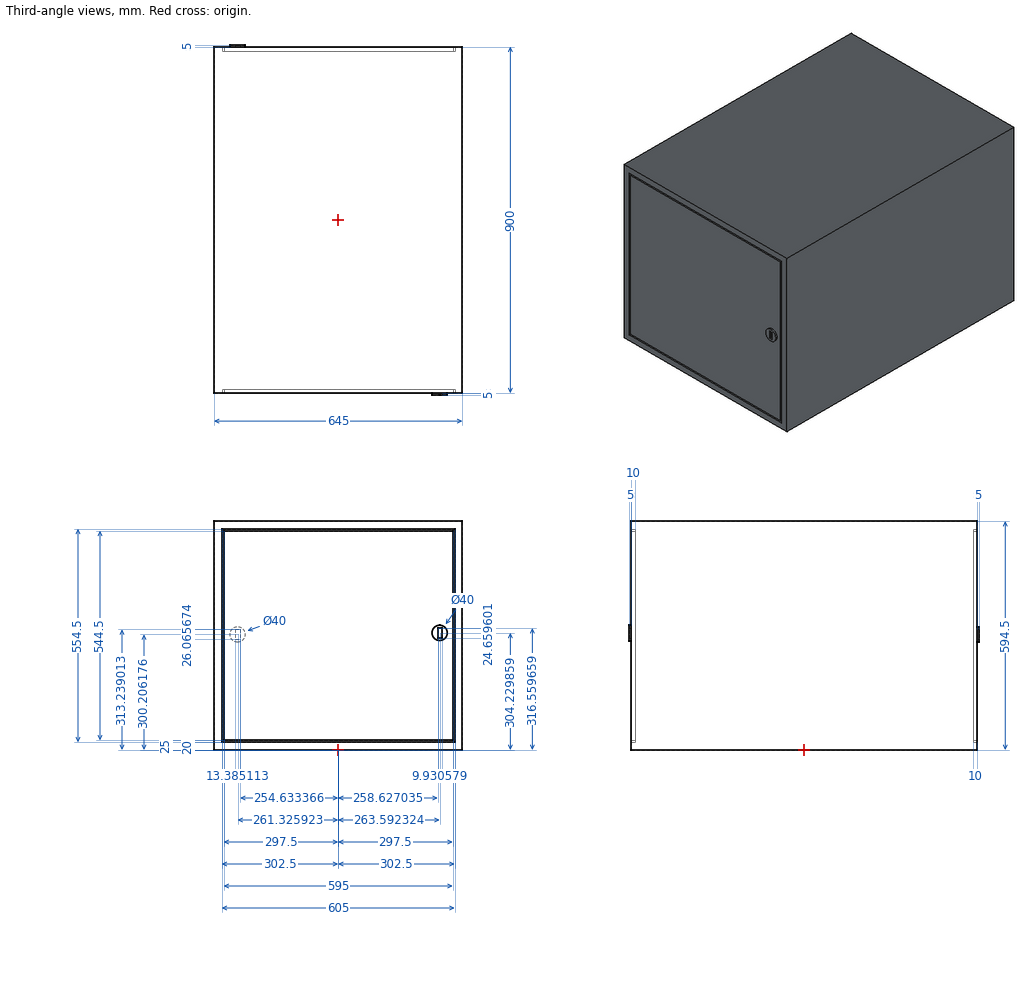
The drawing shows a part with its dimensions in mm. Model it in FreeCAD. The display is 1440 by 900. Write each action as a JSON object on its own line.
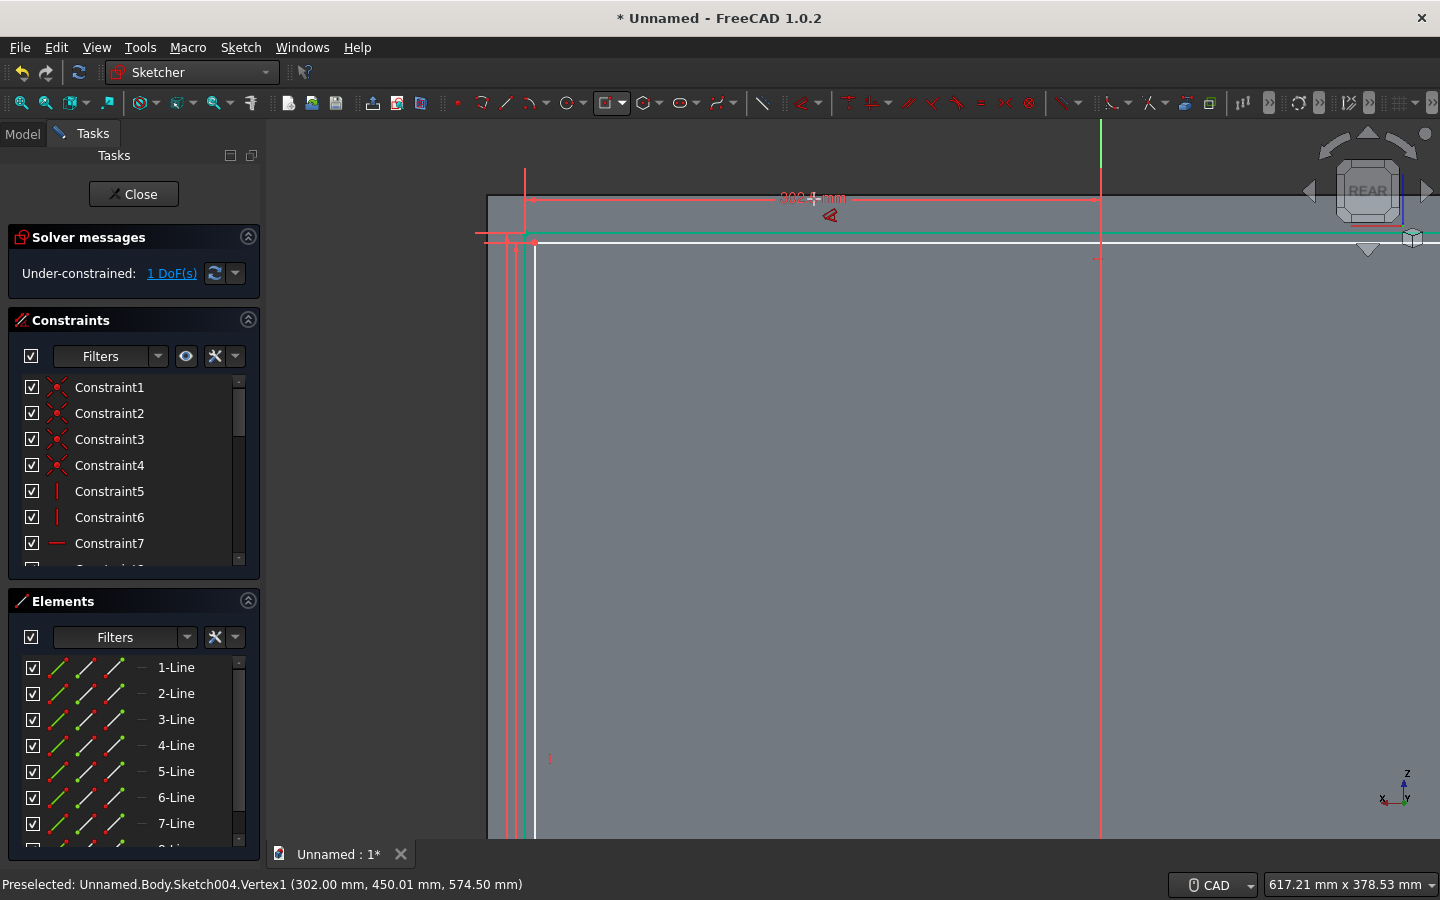
{"action": "left_click", "coordinate": [535, 243]}
{"action": "left_click", "coordinate": [688, 209]}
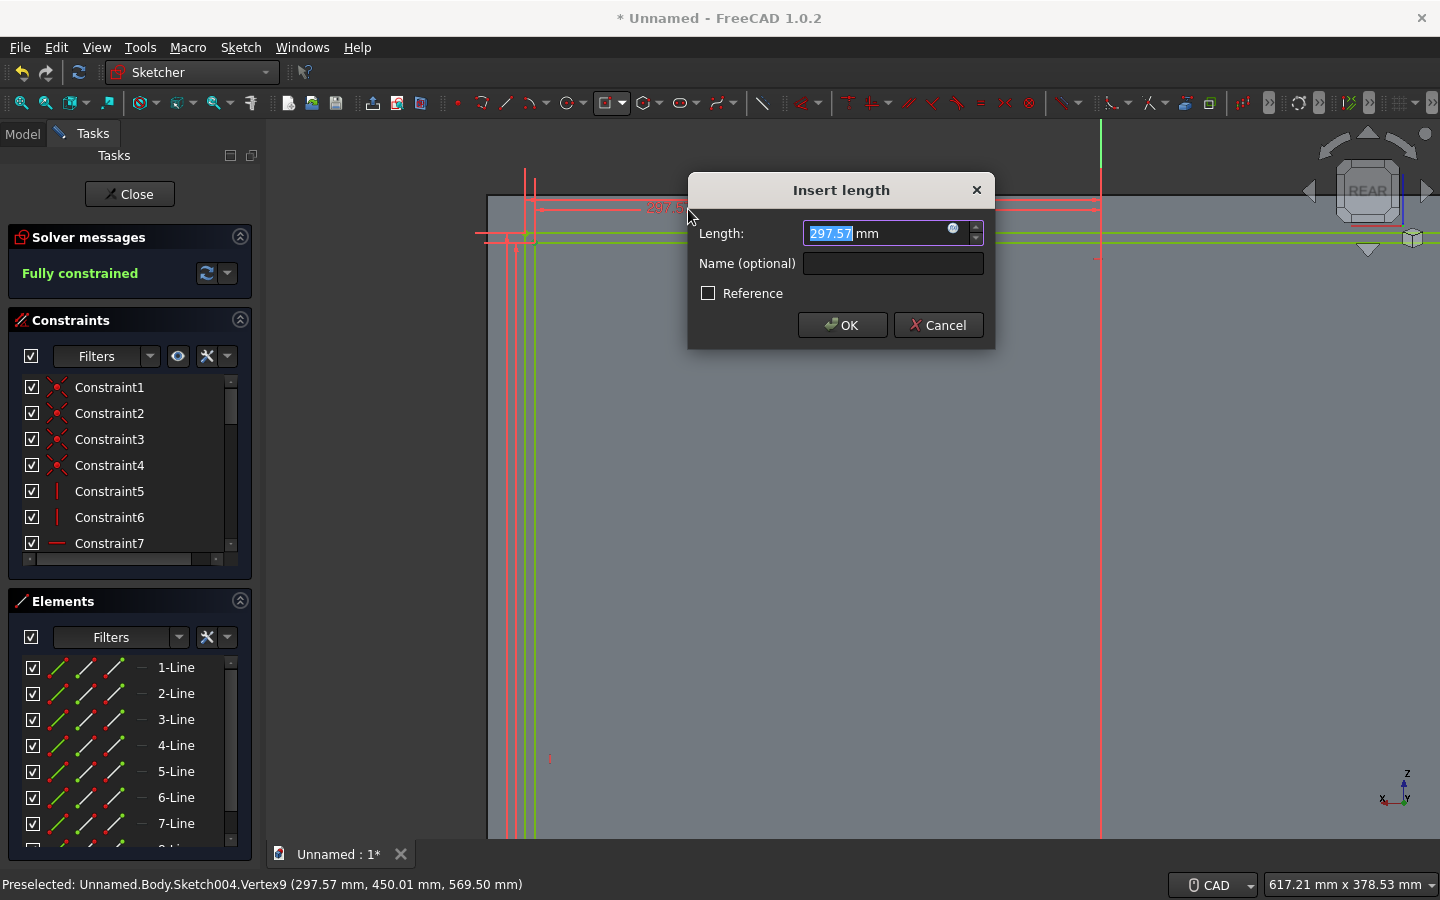
{"action": "type", "text": "297.5"}
{"action": "key", "text": "Return"}
{"action": "key", "text": "Escape"}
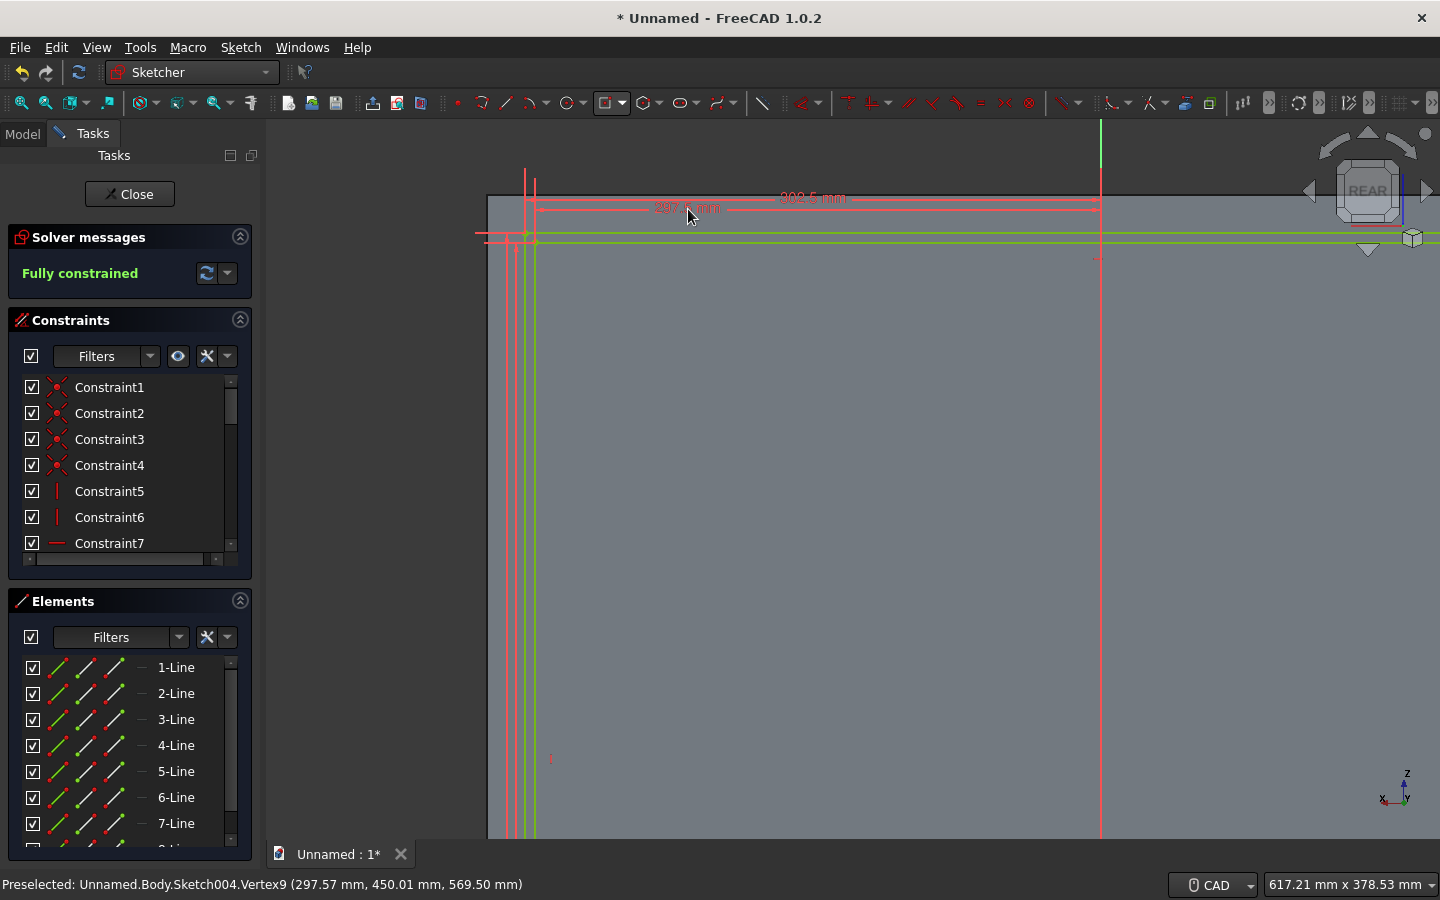
{"action": "left_click", "coordinate": [130, 194]}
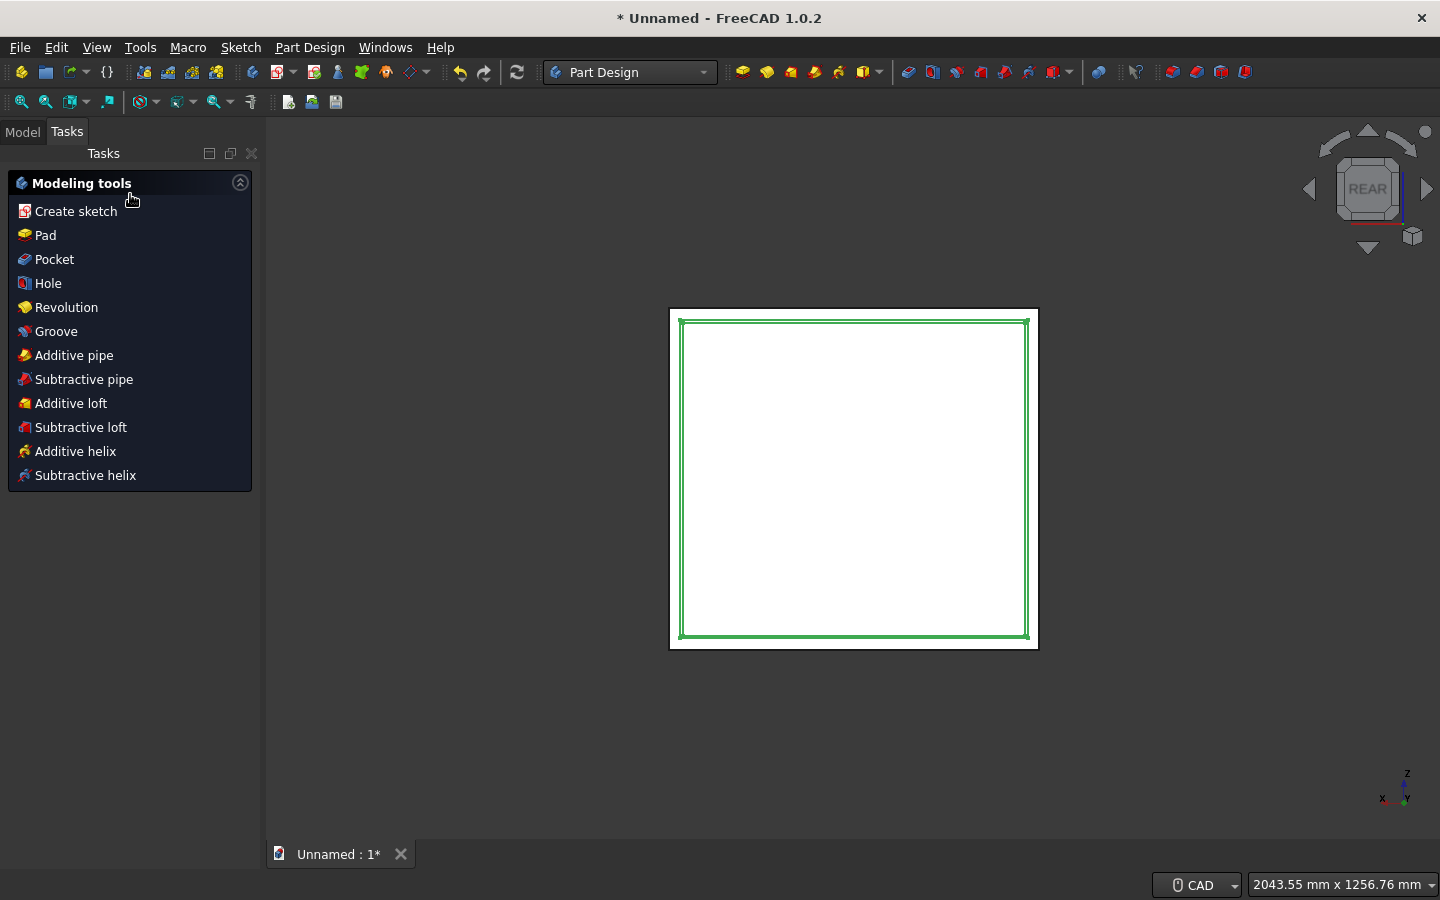
{"action": "left_click", "coordinate": [910, 72]}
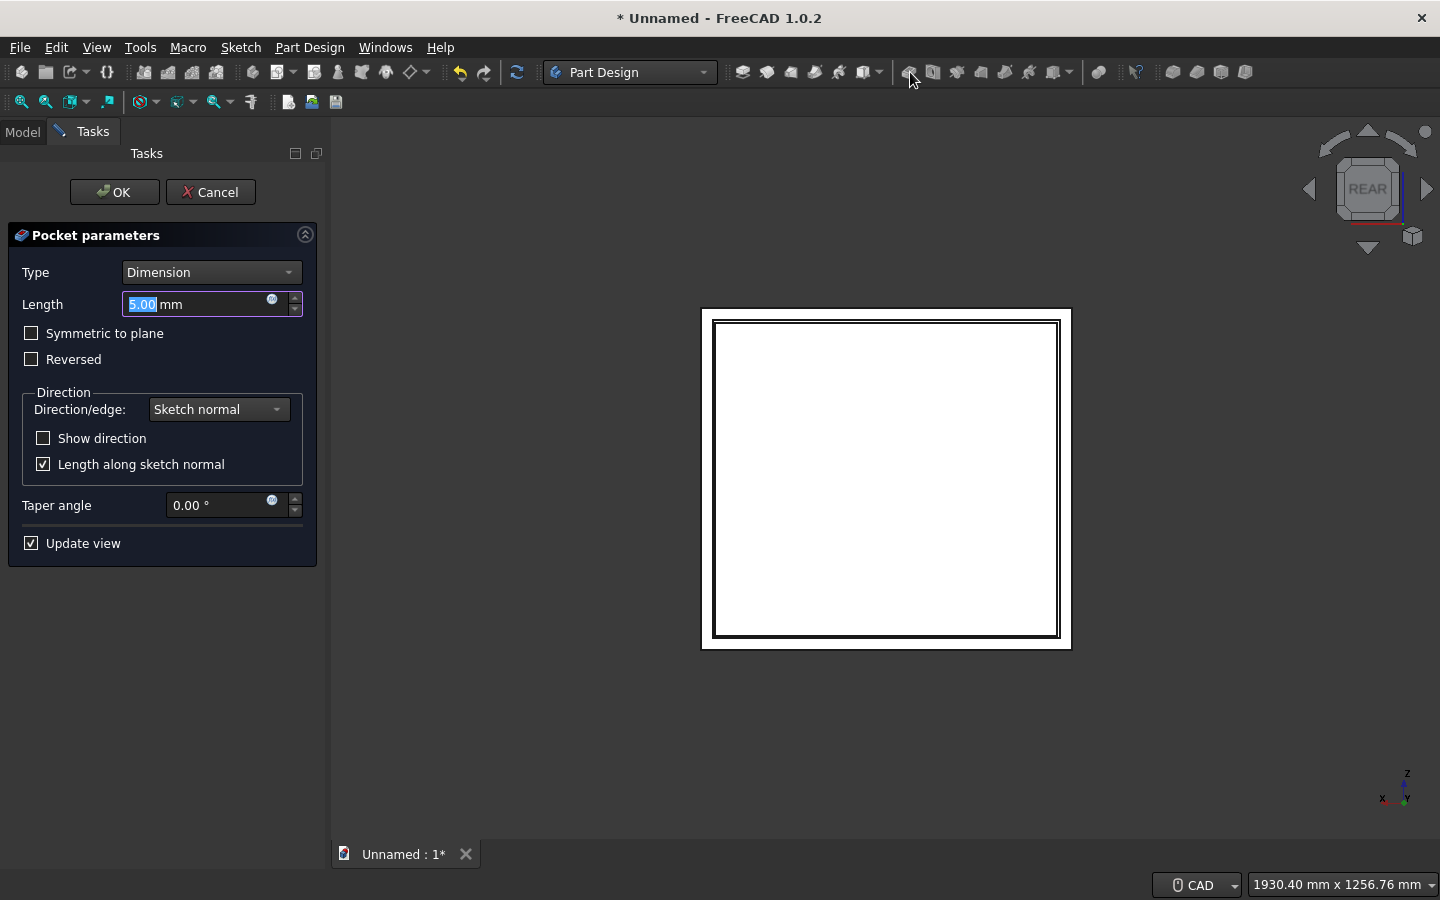
{"action": "type", "text": "10"}
{"action": "key", "text": "Tab"}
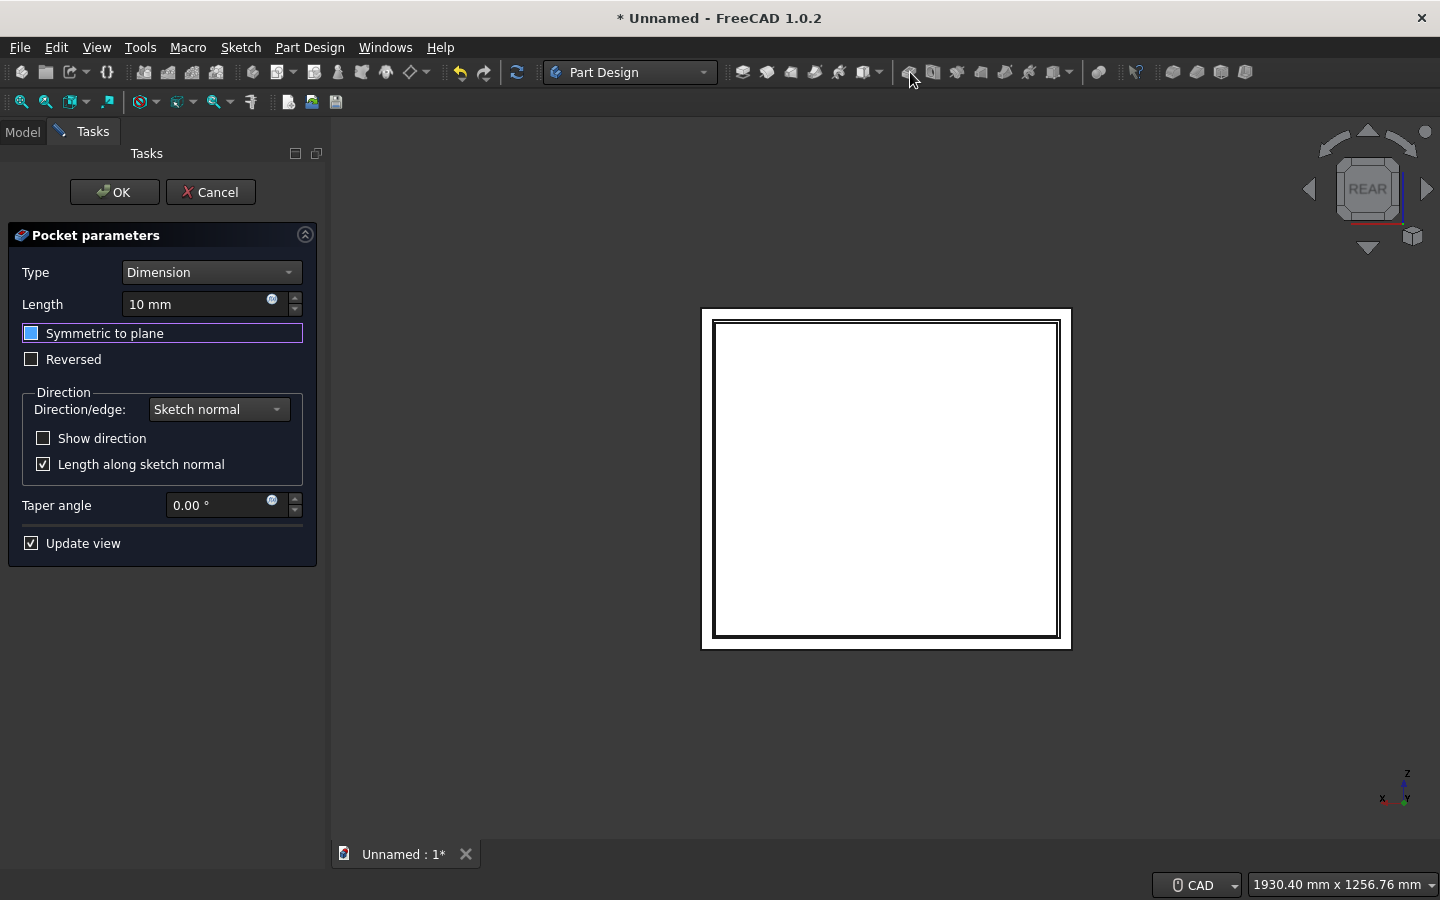
{"action": "left_click", "coordinate": [115, 192]}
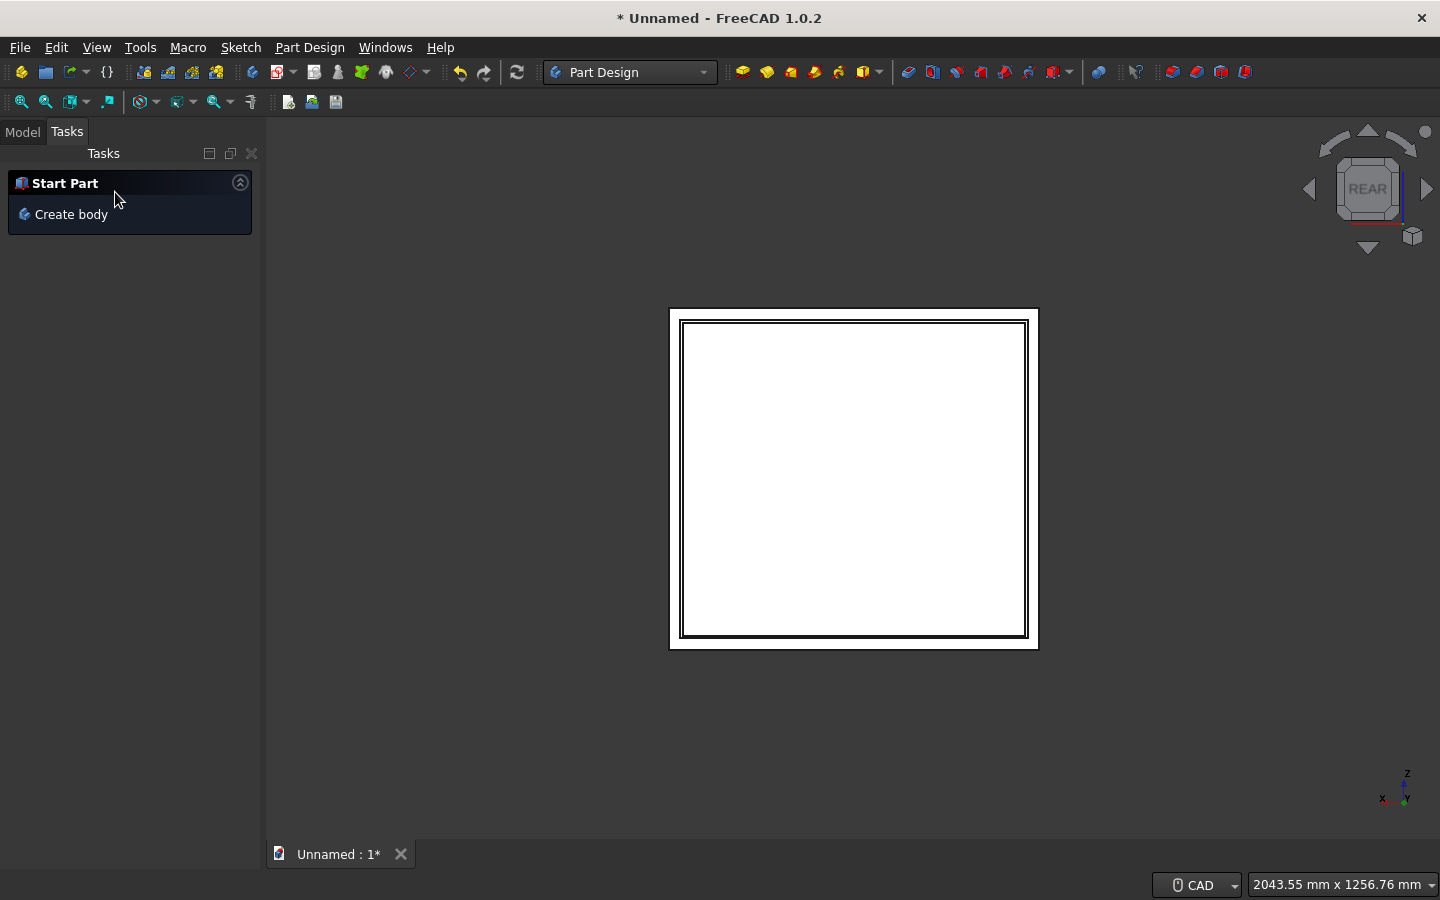
{"action": "left_click", "coordinate": [854, 478]}